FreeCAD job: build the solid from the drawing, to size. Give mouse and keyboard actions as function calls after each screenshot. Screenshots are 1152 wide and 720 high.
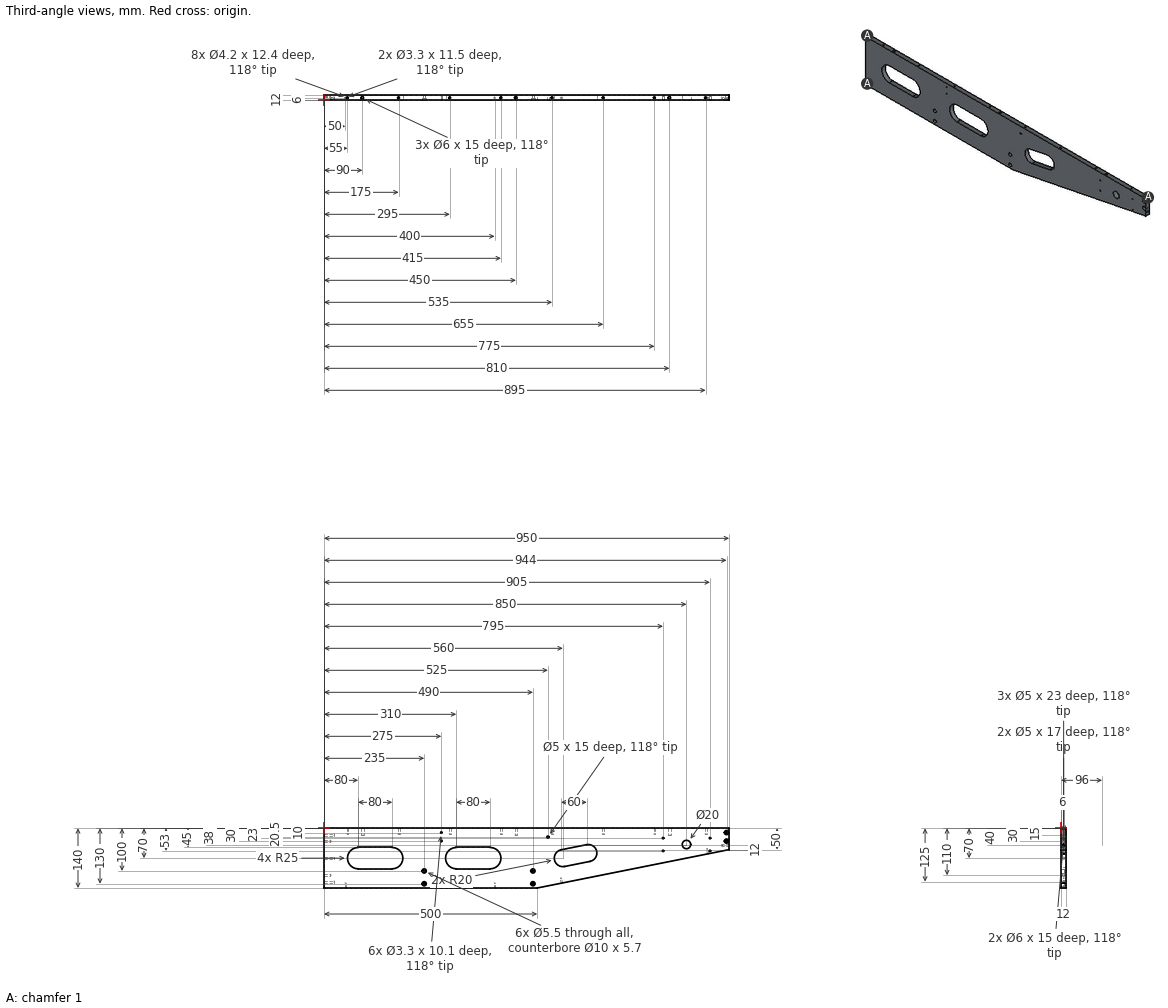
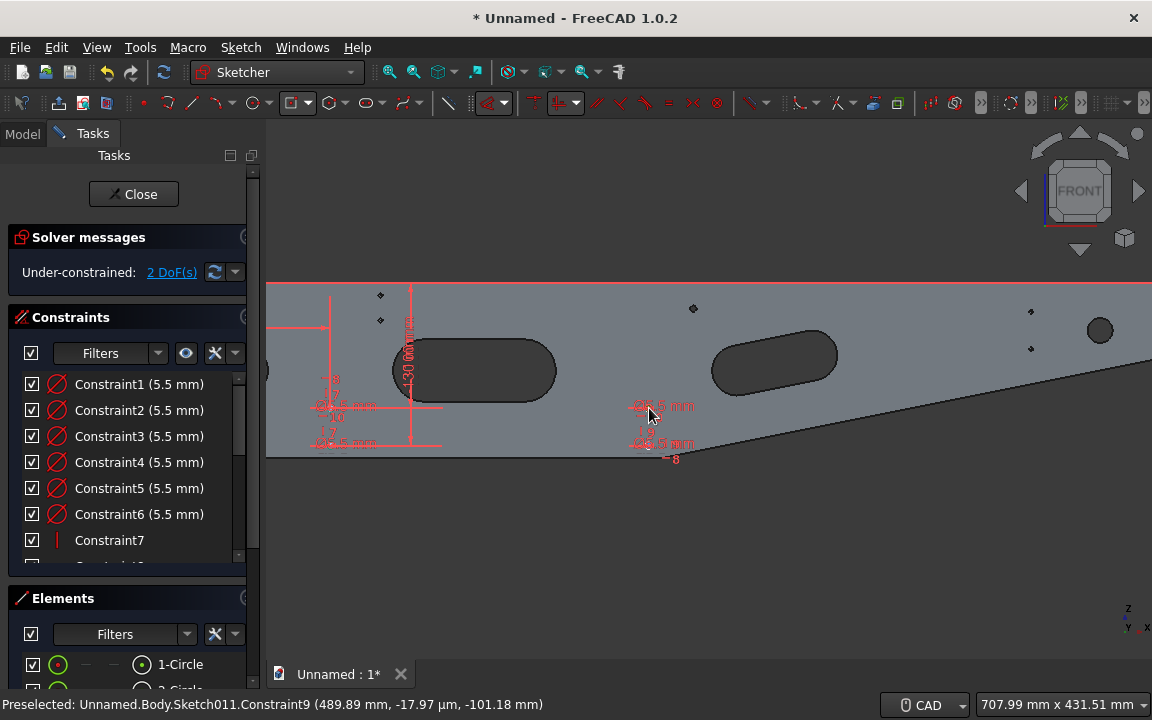
key(l)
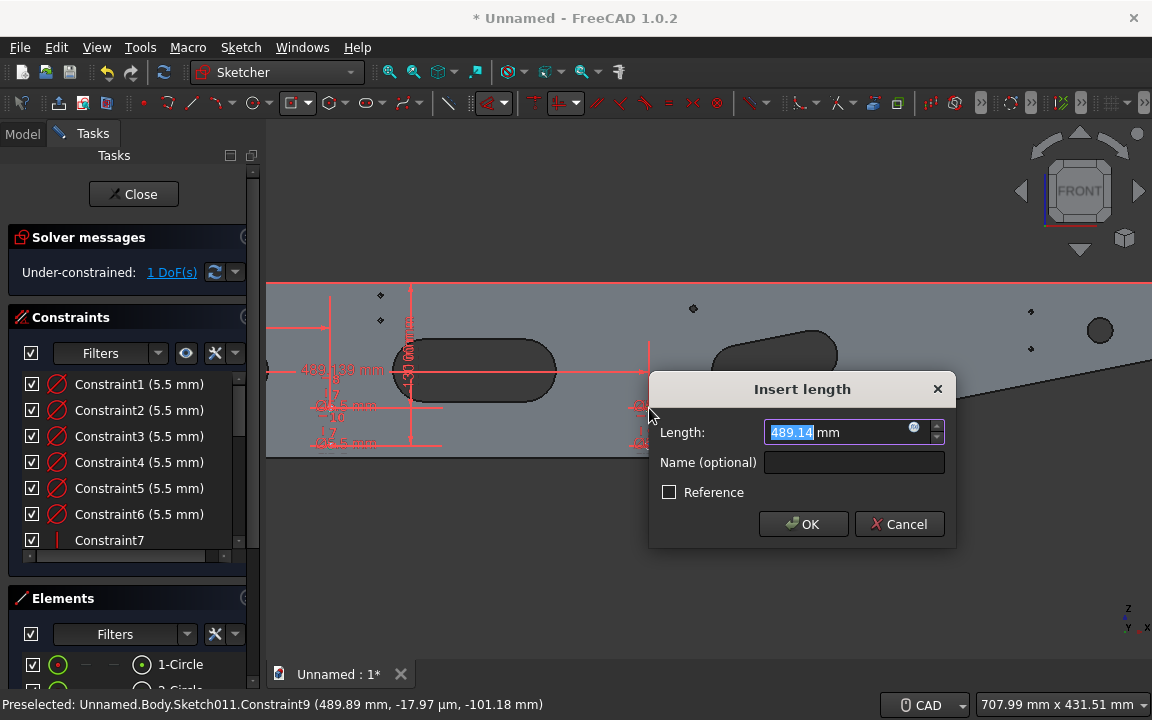
text(490)
key(Return)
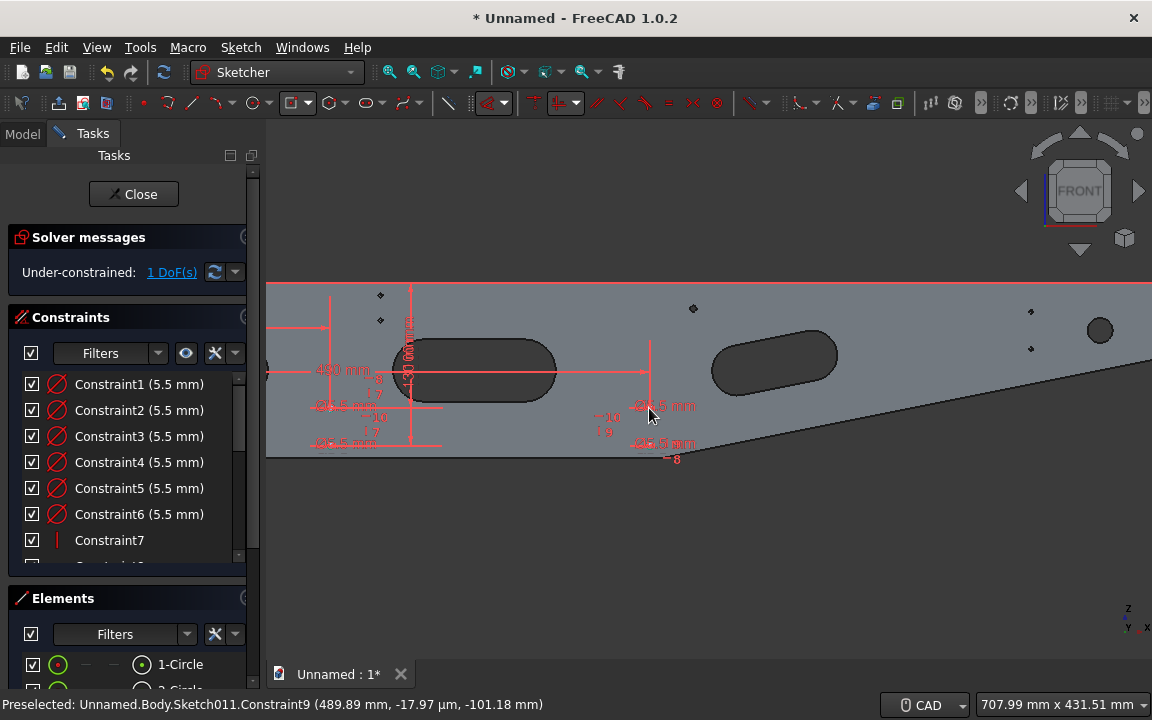
scroll(650, 408, down, 4)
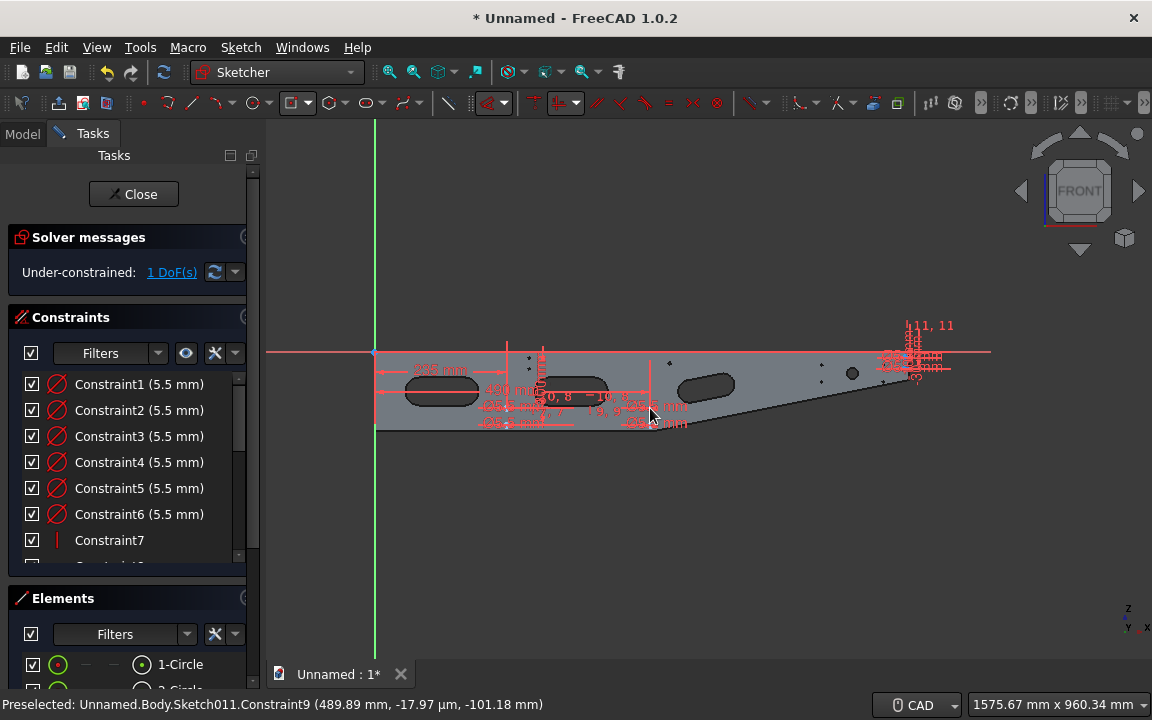
click(905, 358)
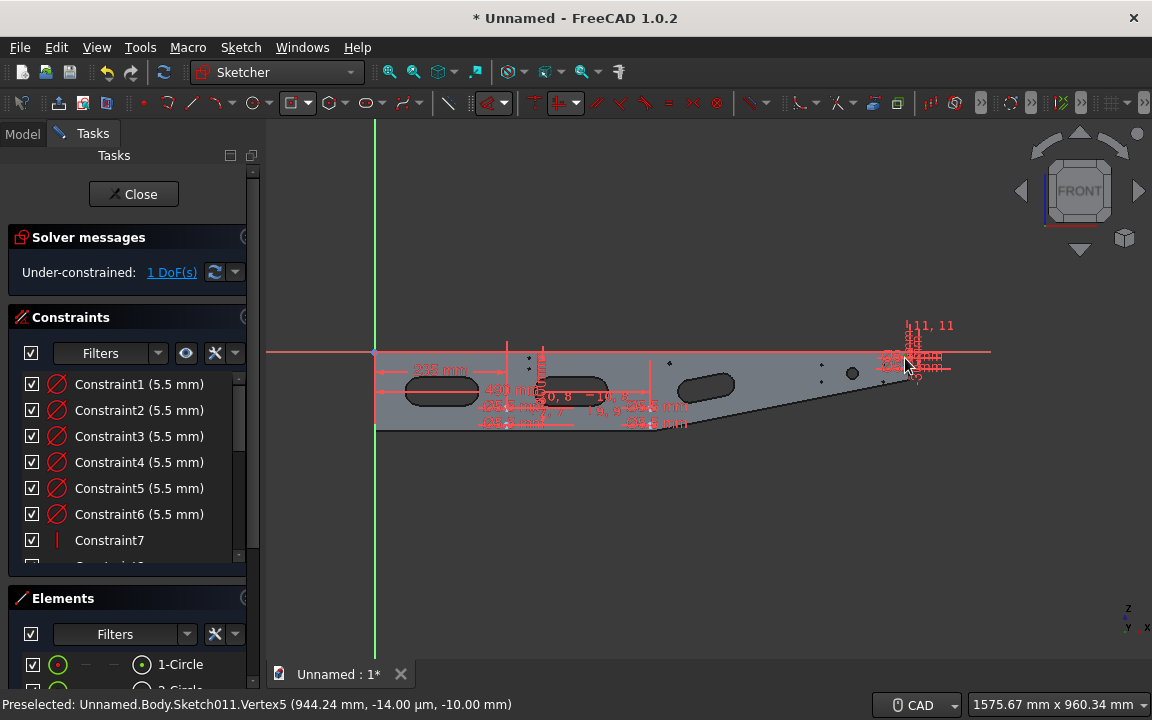
key(l)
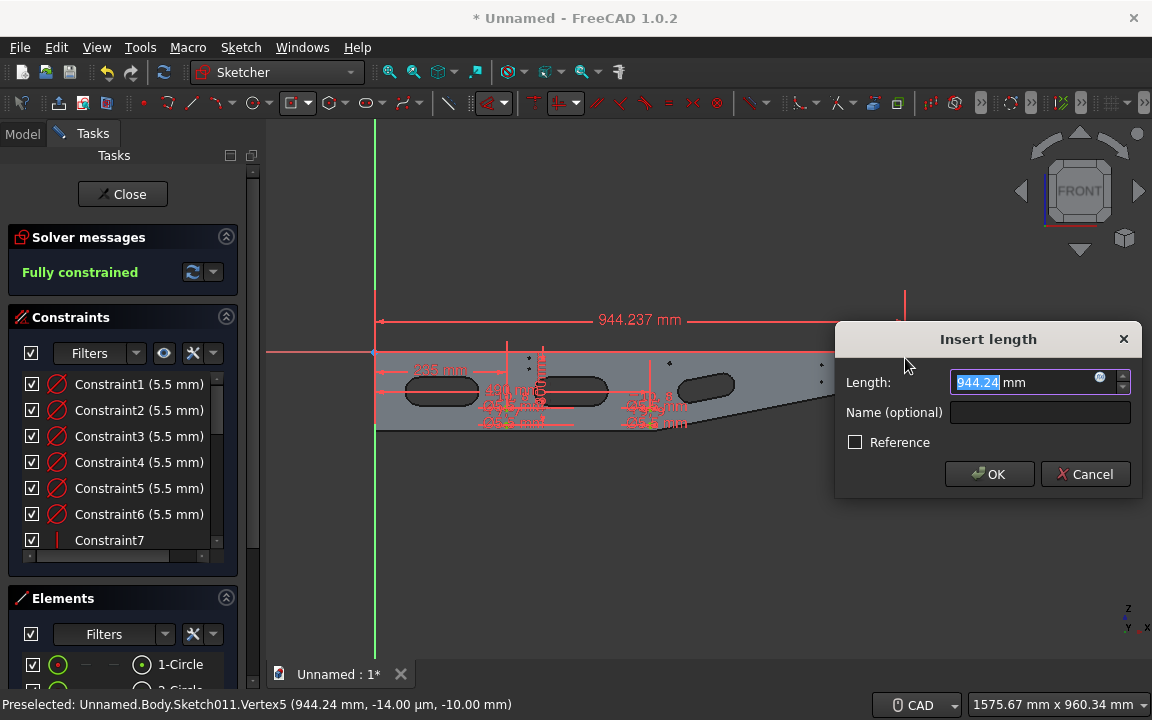
text(944)
key(Return)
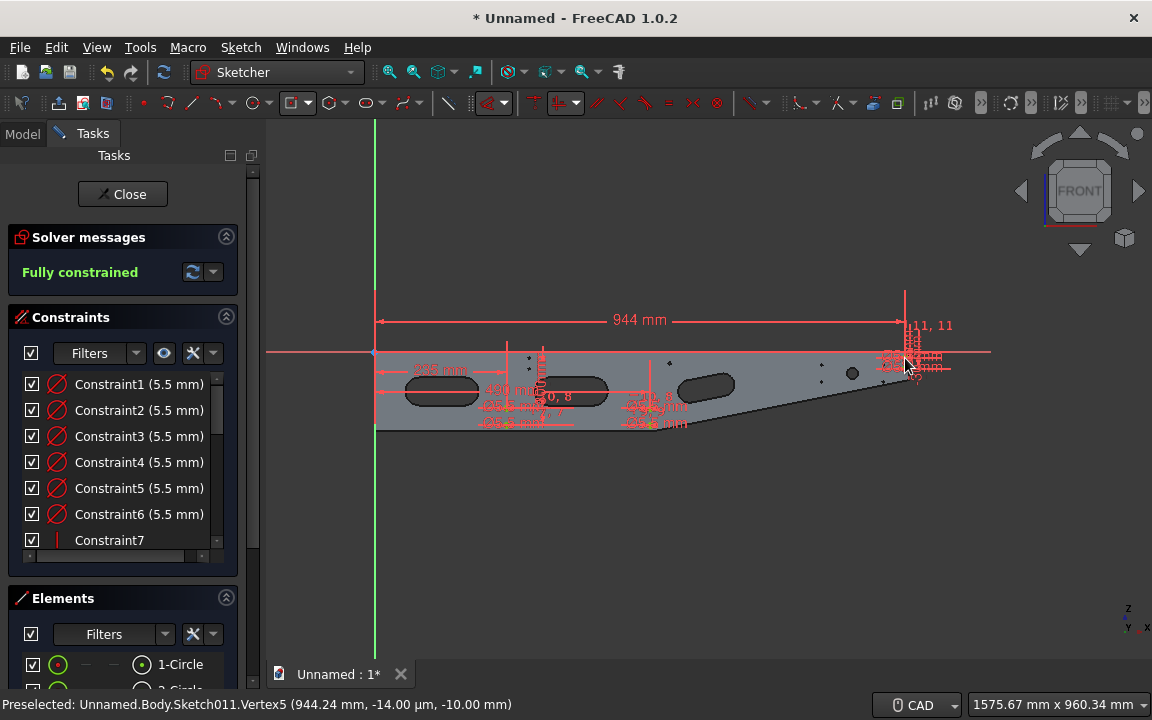
click(123, 194)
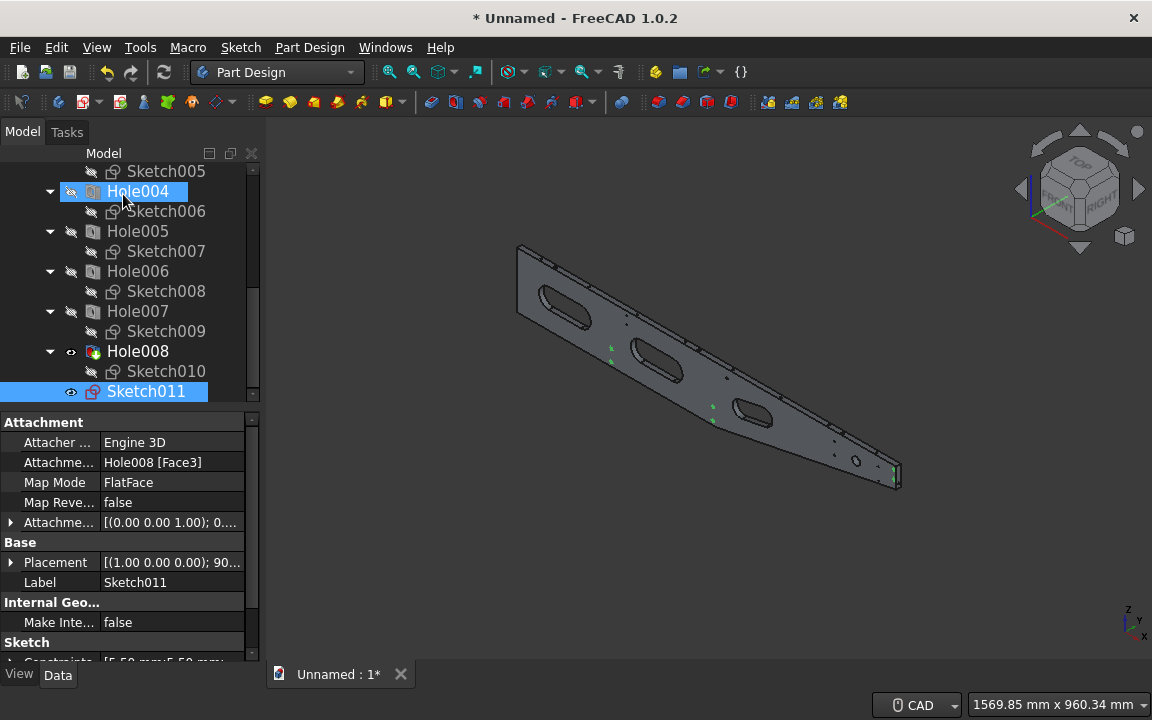
click(456, 102)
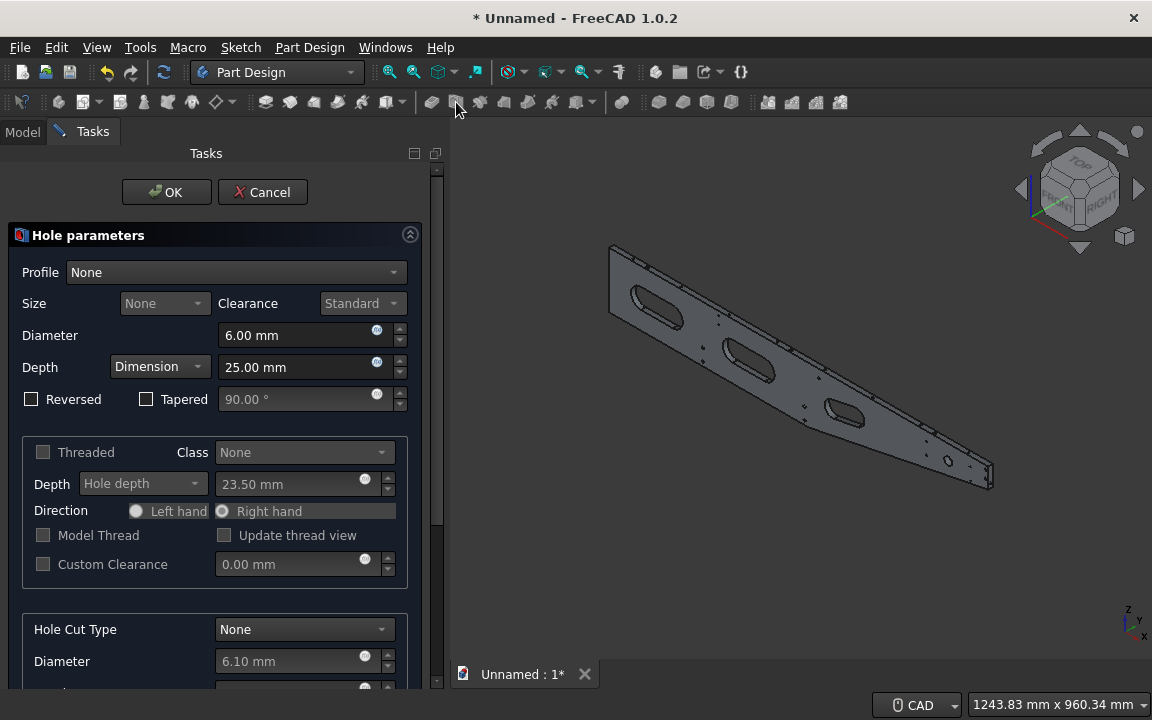
triple_click(305, 335)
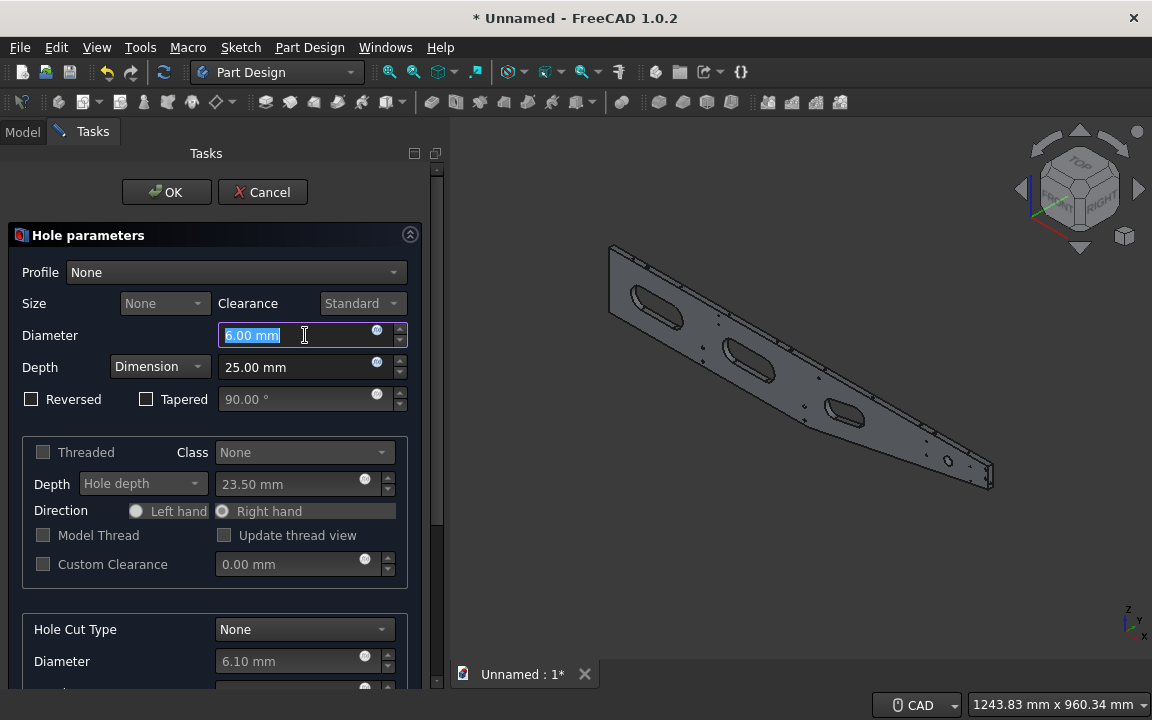
text(5.5)
key(Tab)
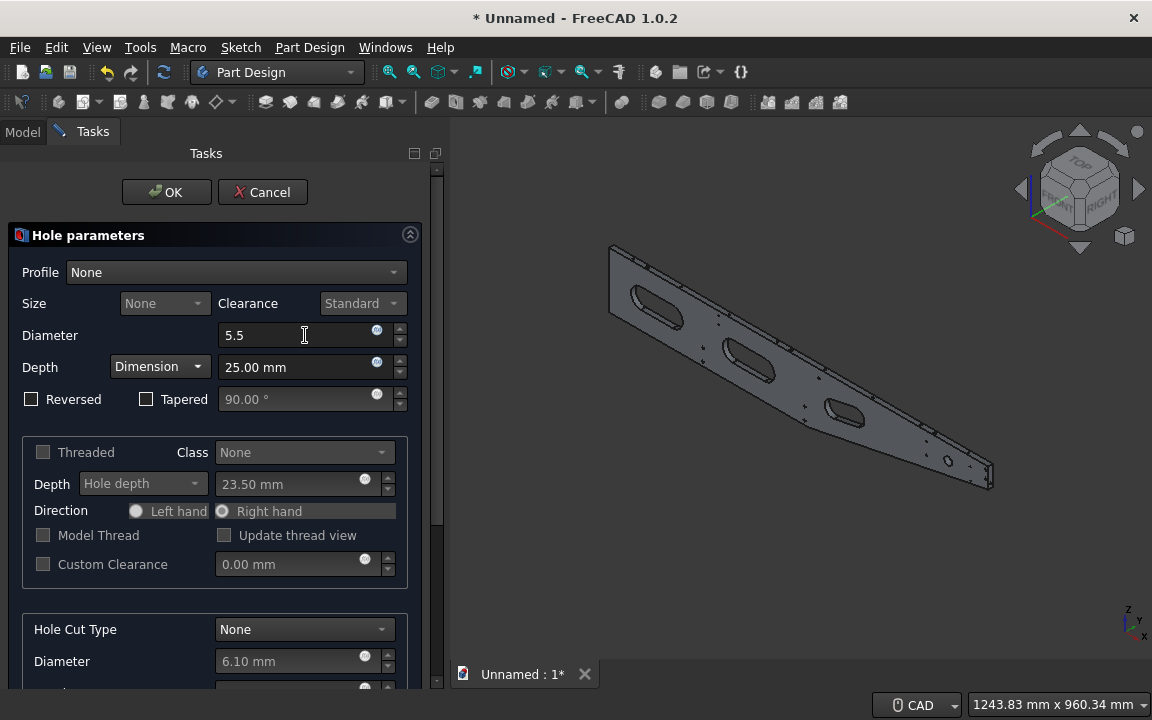
click(161, 366)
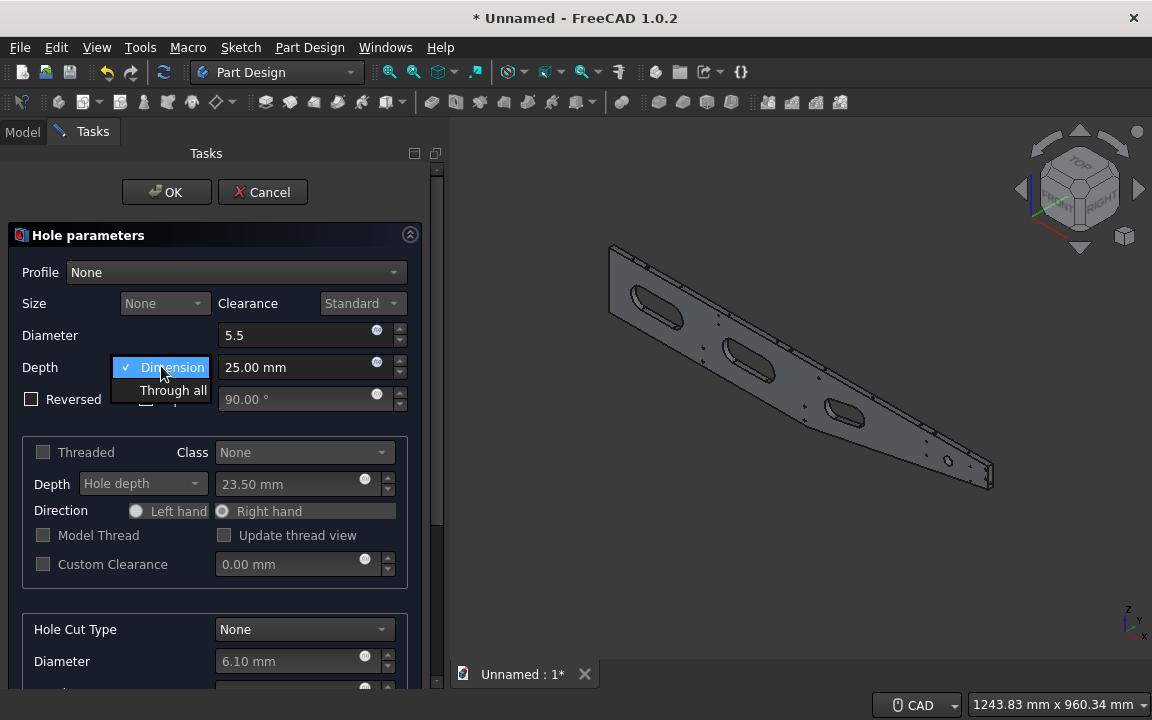
click(160, 390)